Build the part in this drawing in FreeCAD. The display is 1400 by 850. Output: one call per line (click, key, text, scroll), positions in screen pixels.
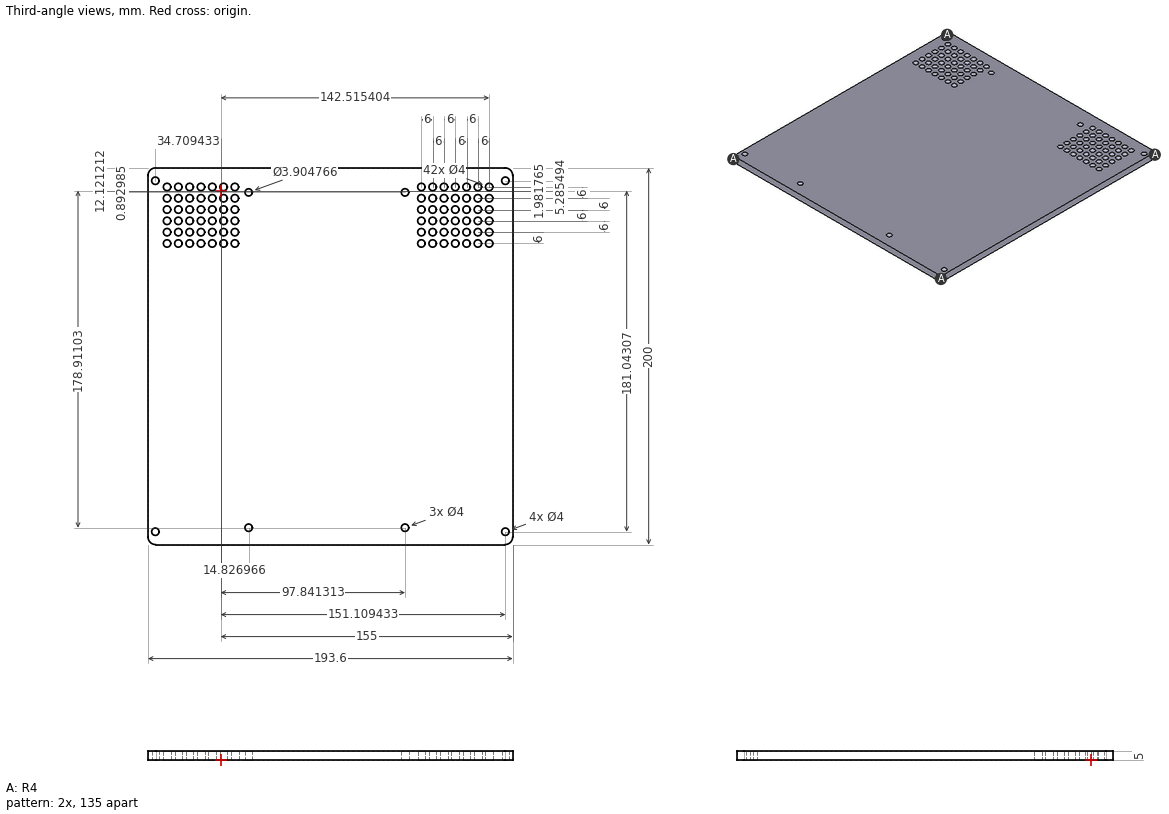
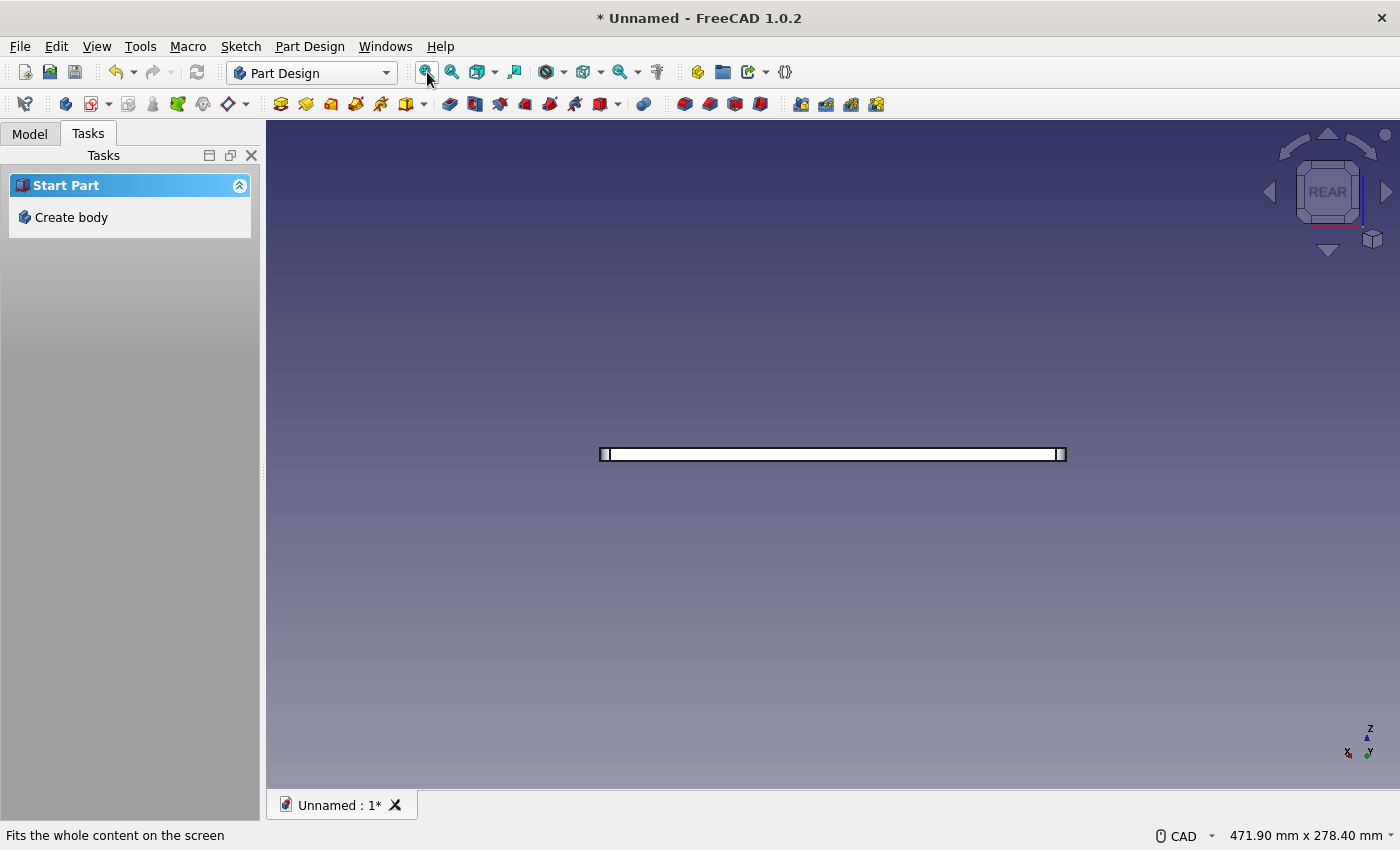
key(0)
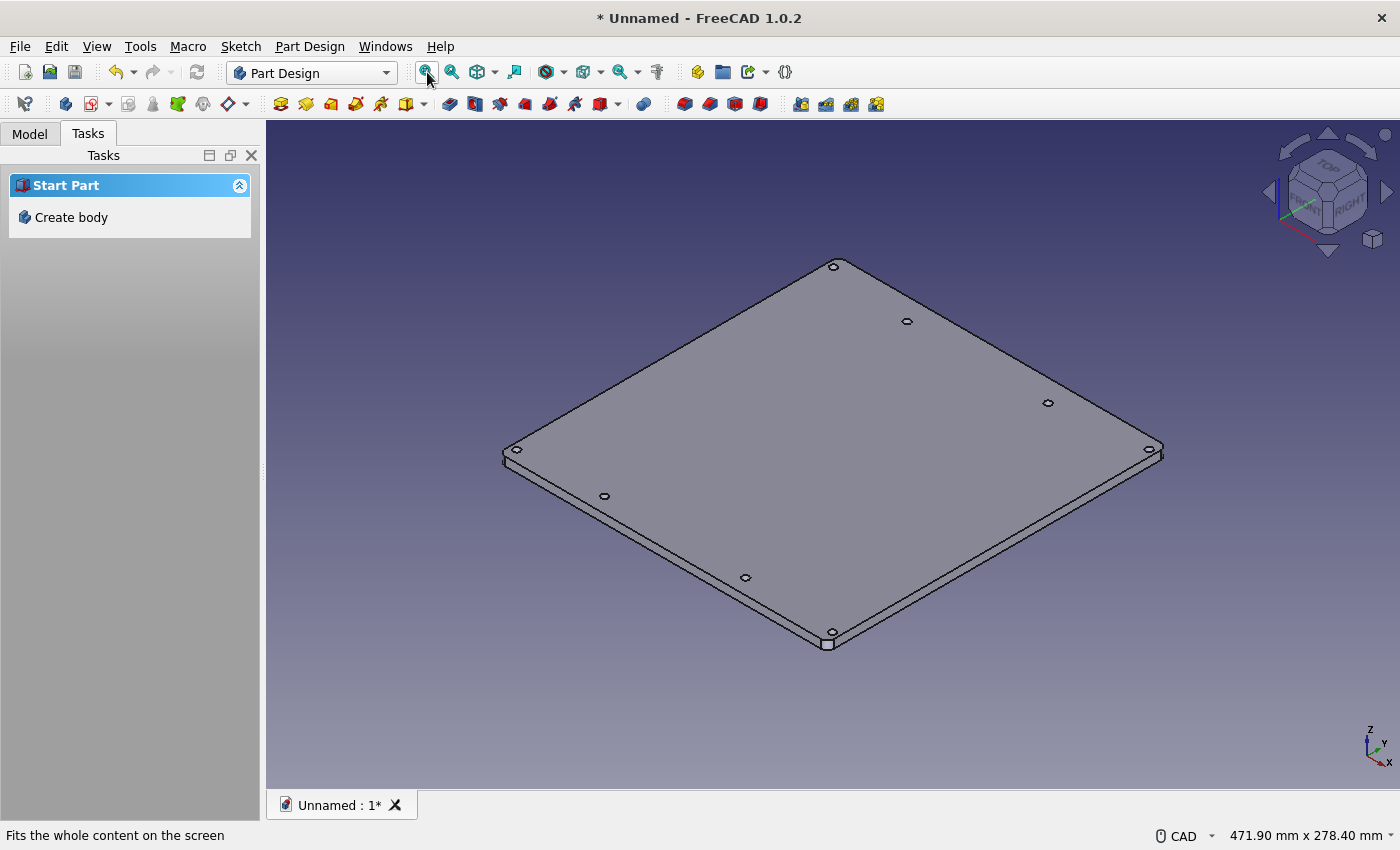
click(833, 449)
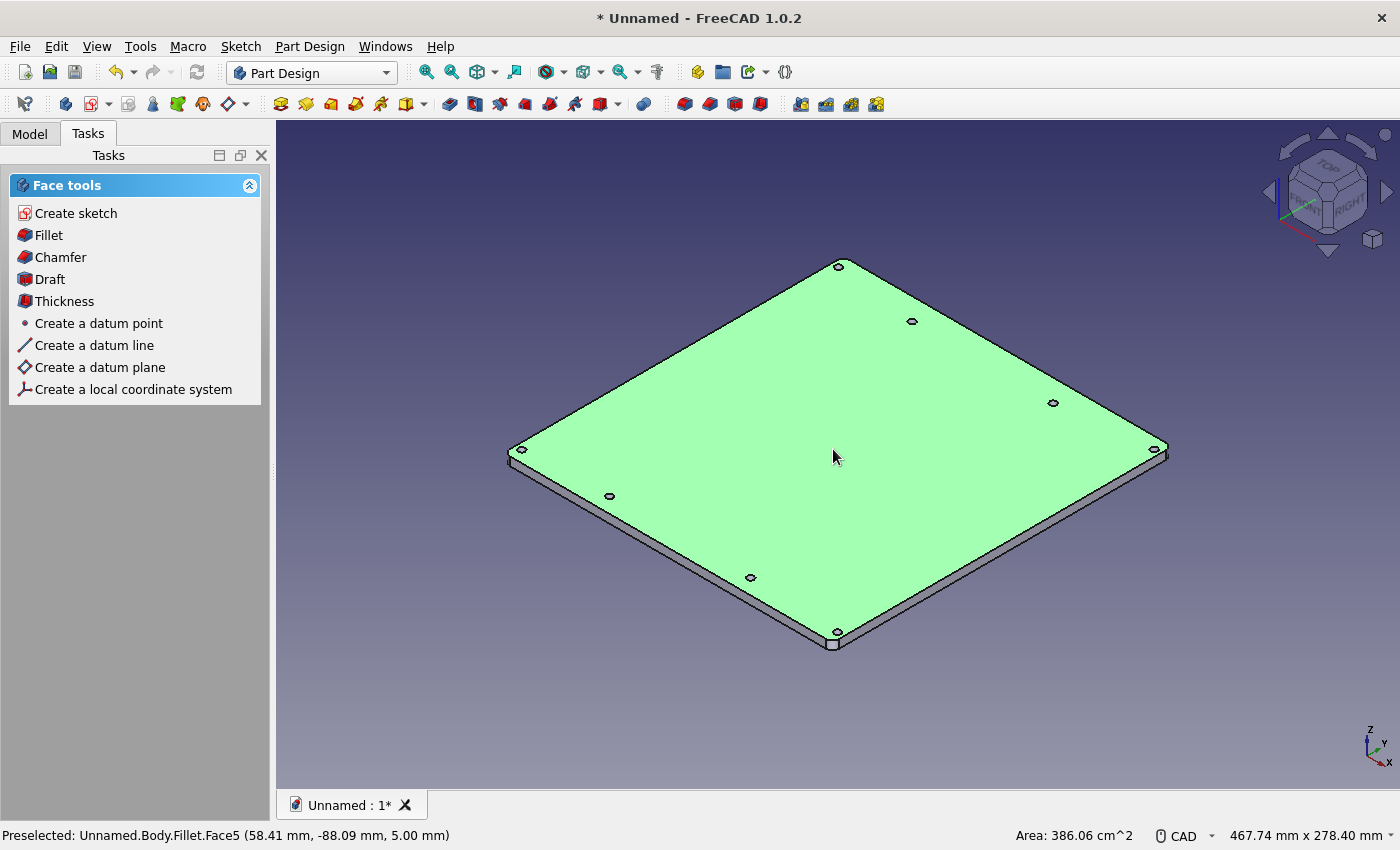
click(90, 104)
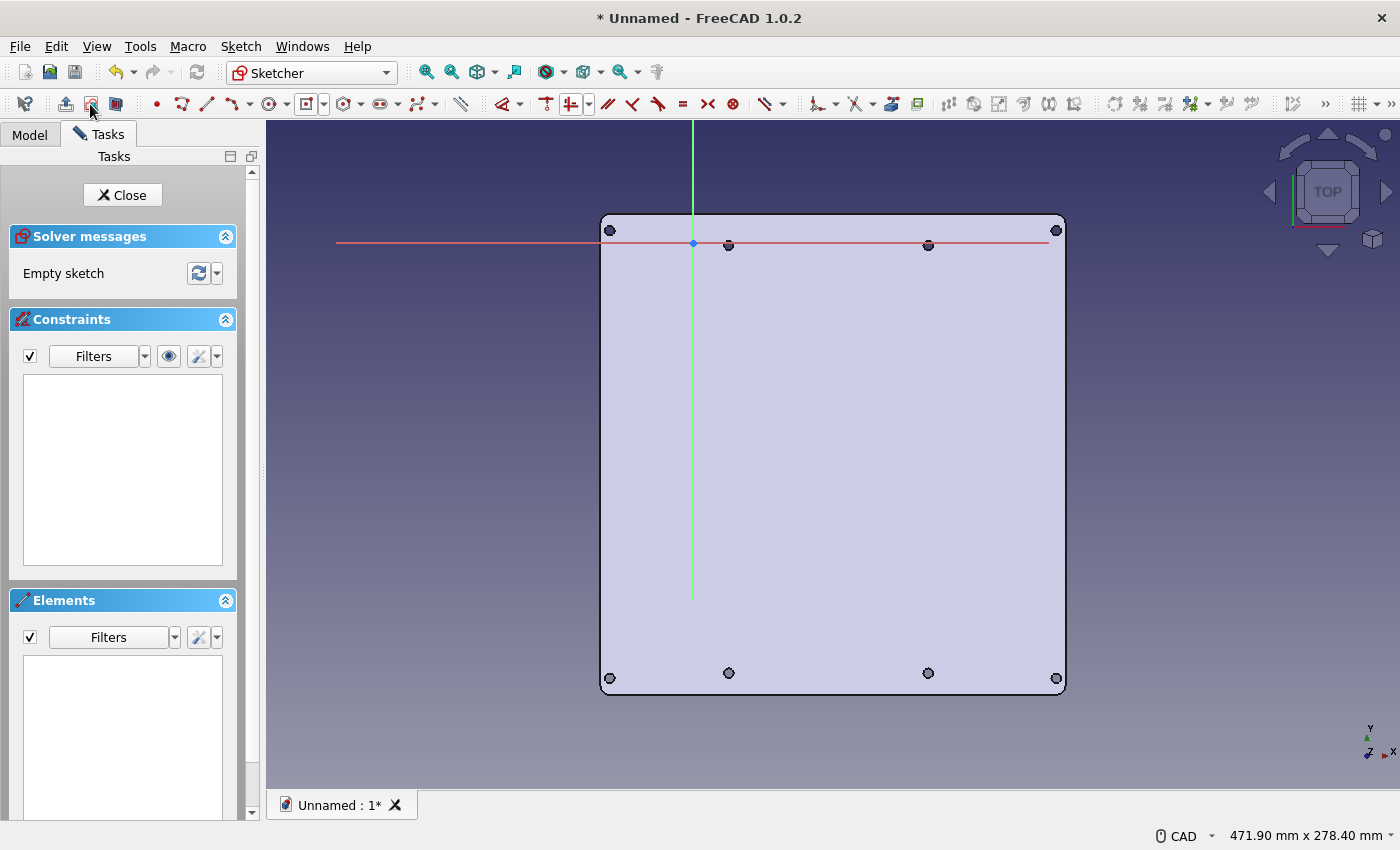
scroll(1050, 229, up, 8)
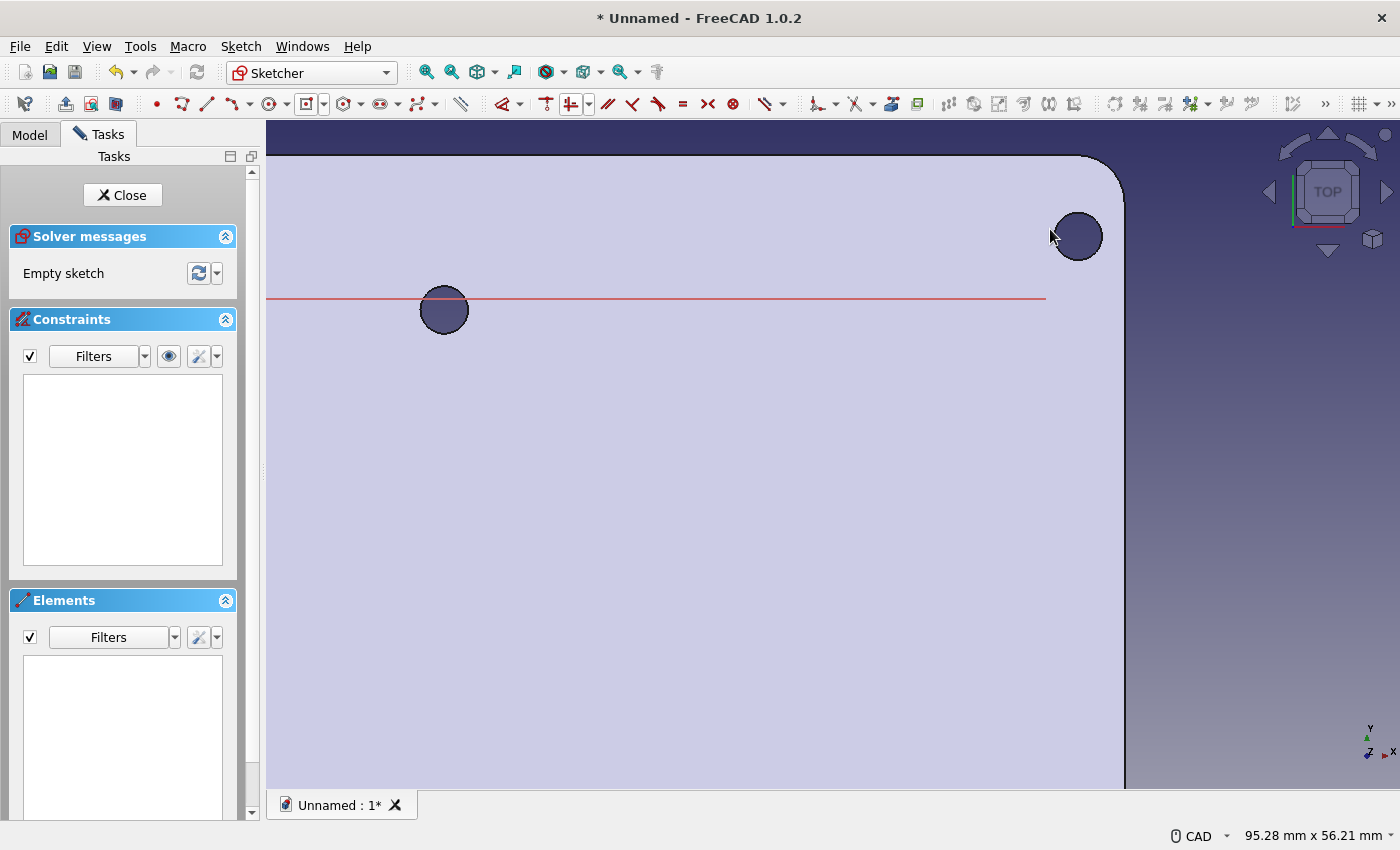
click(268, 104)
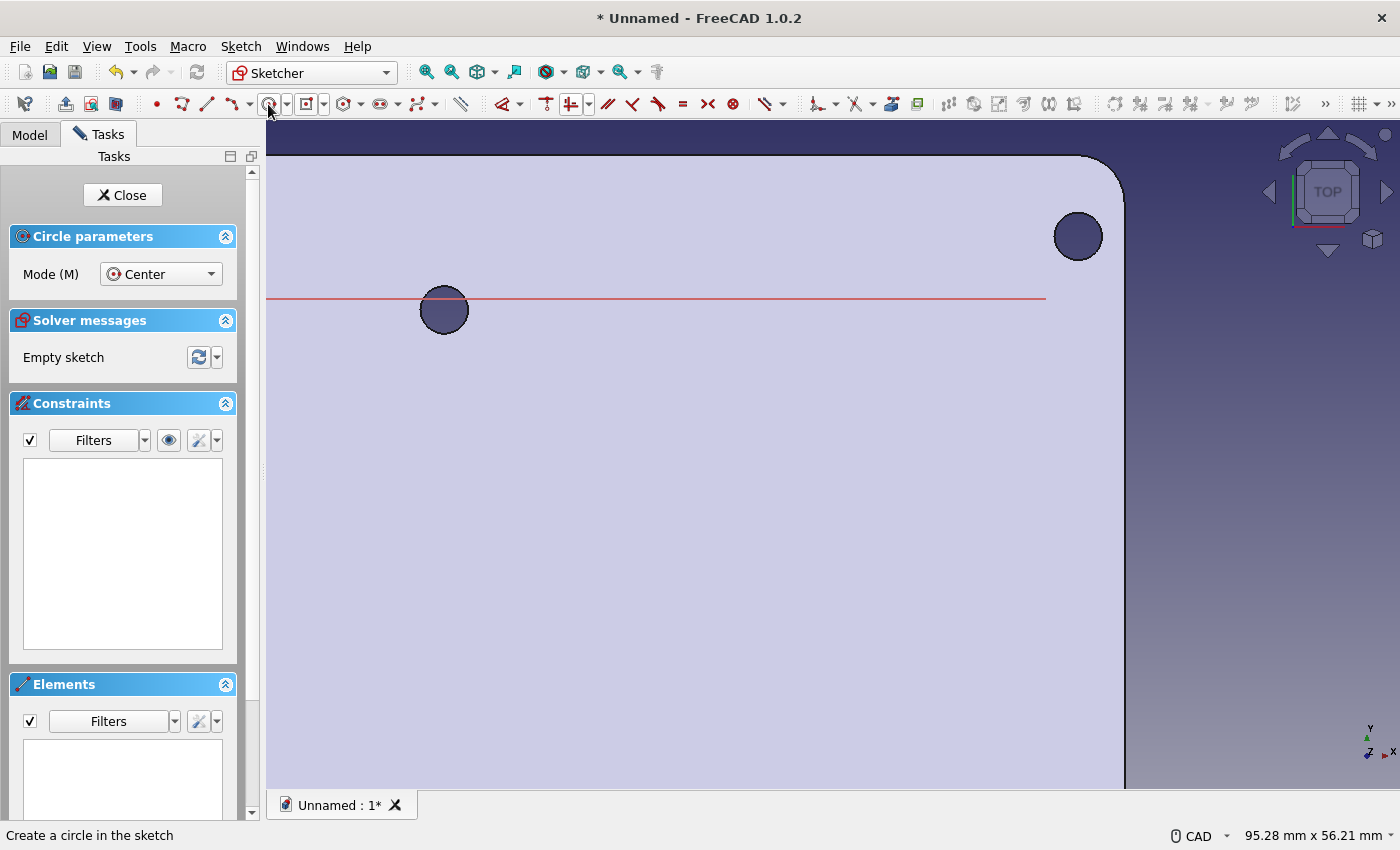
click(976, 276)
move(993, 259)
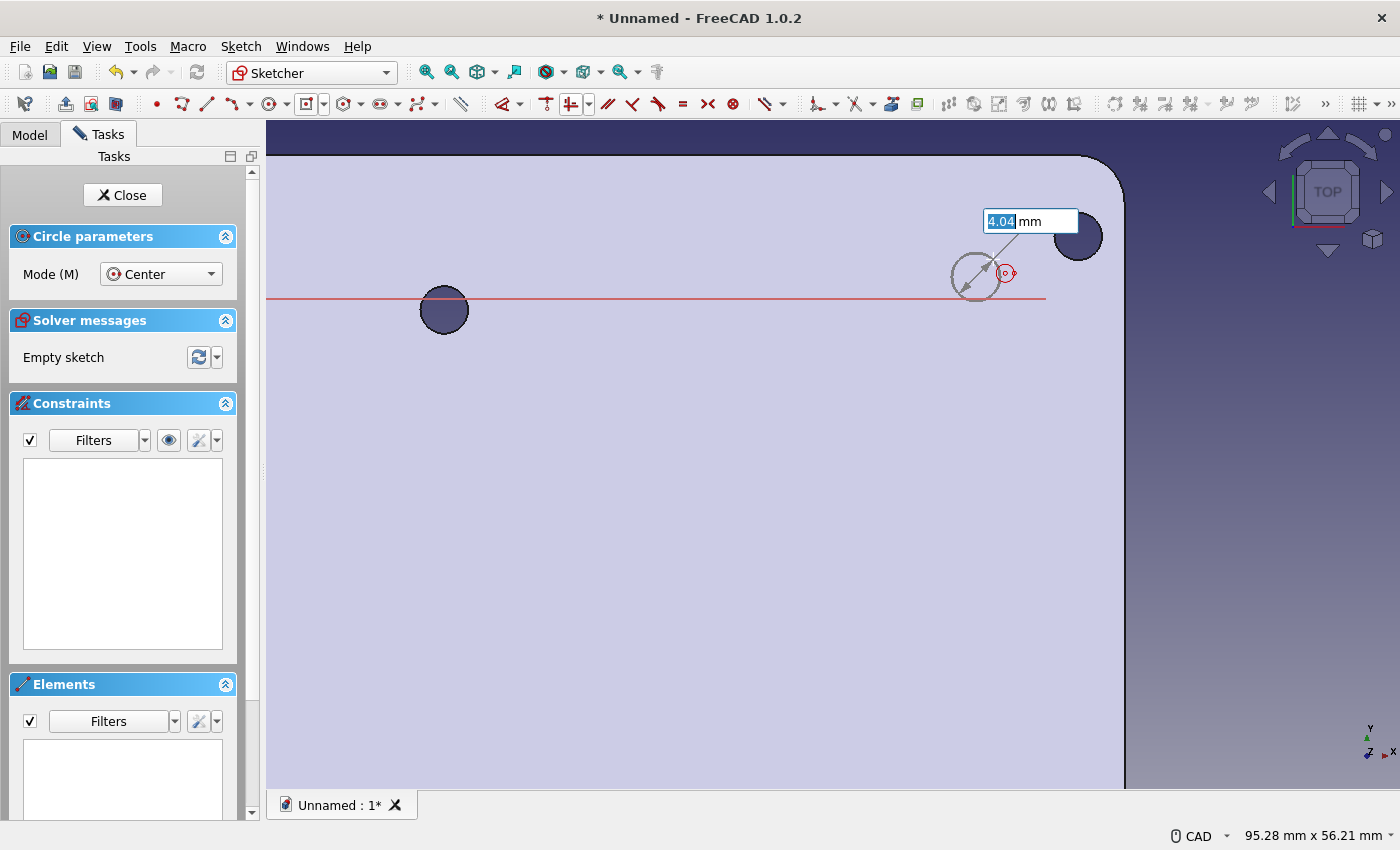
text(4)
key(Return)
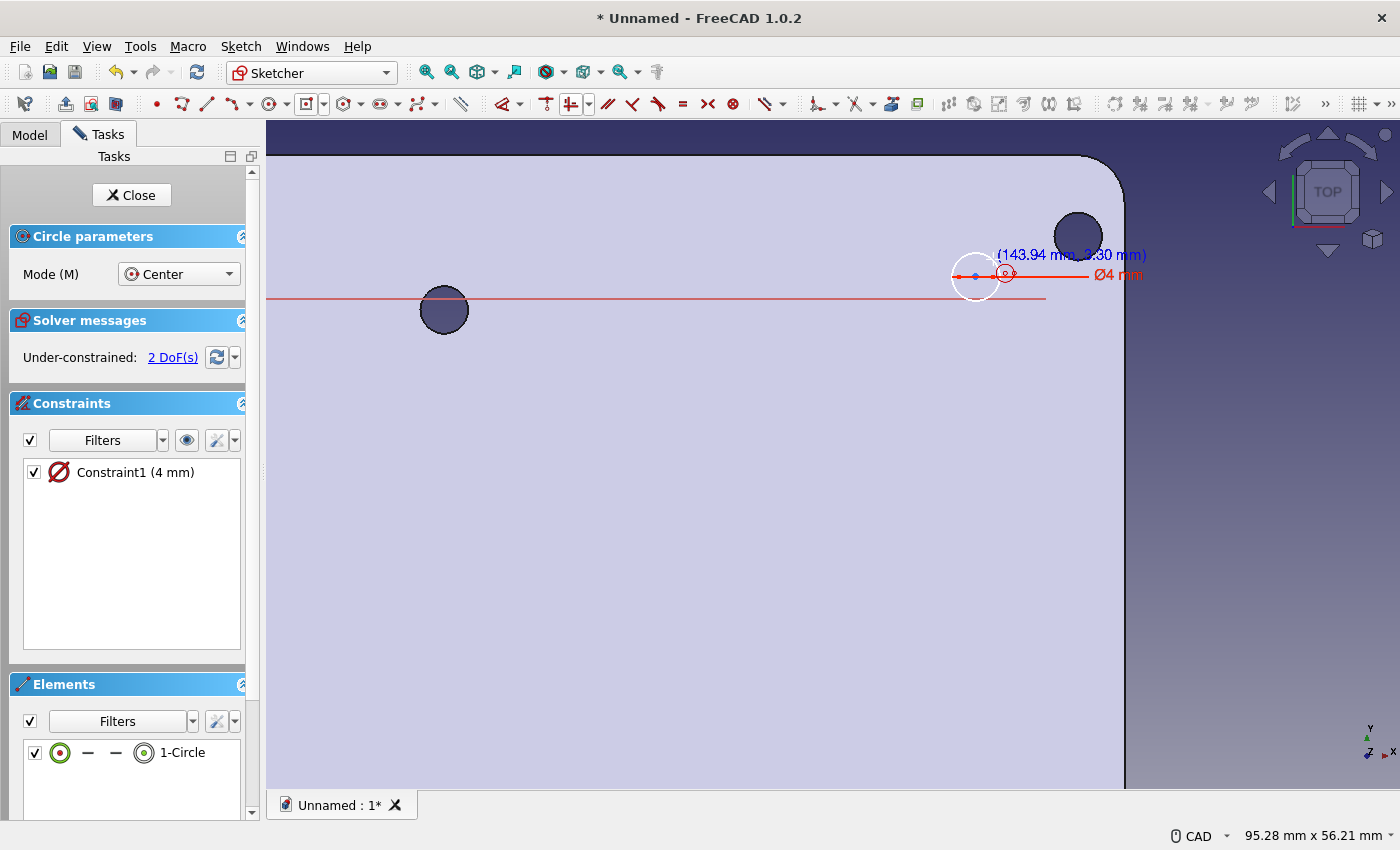
click(905, 276)
move(921, 259)